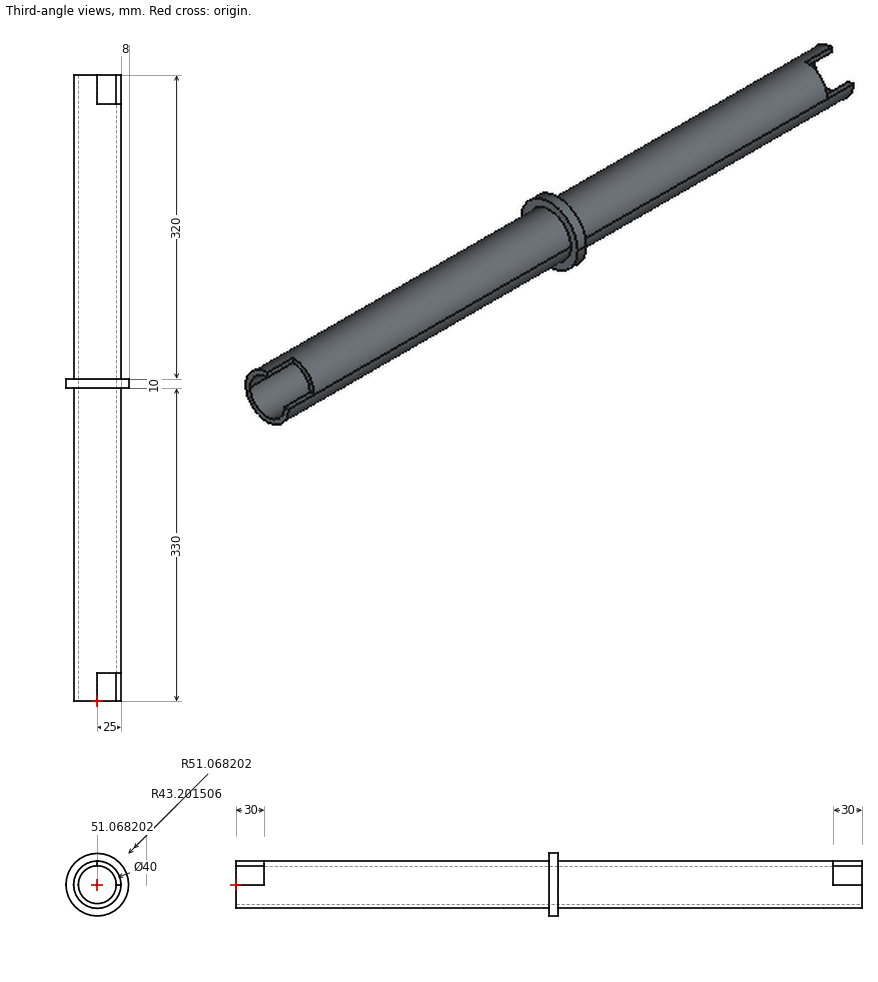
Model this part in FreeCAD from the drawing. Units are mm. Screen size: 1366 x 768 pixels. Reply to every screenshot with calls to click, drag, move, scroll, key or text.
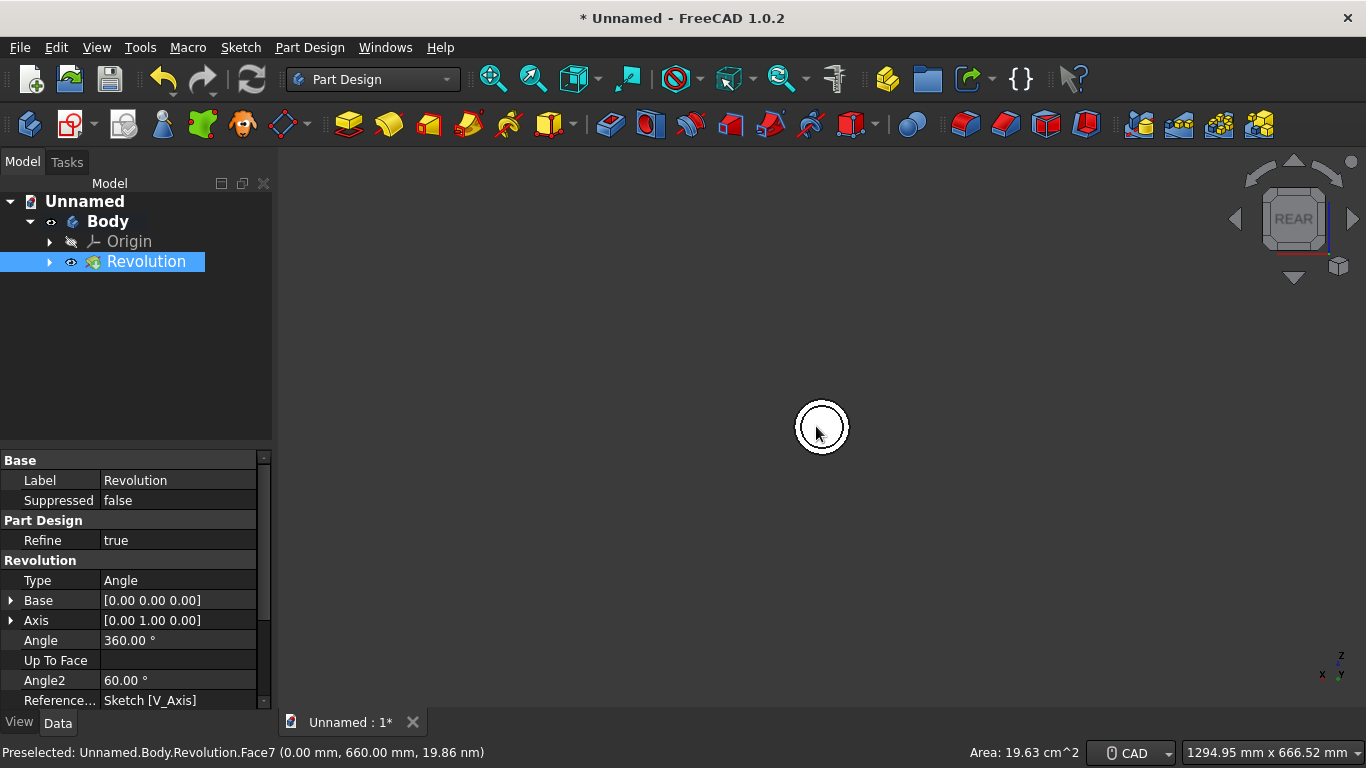
click(70, 124)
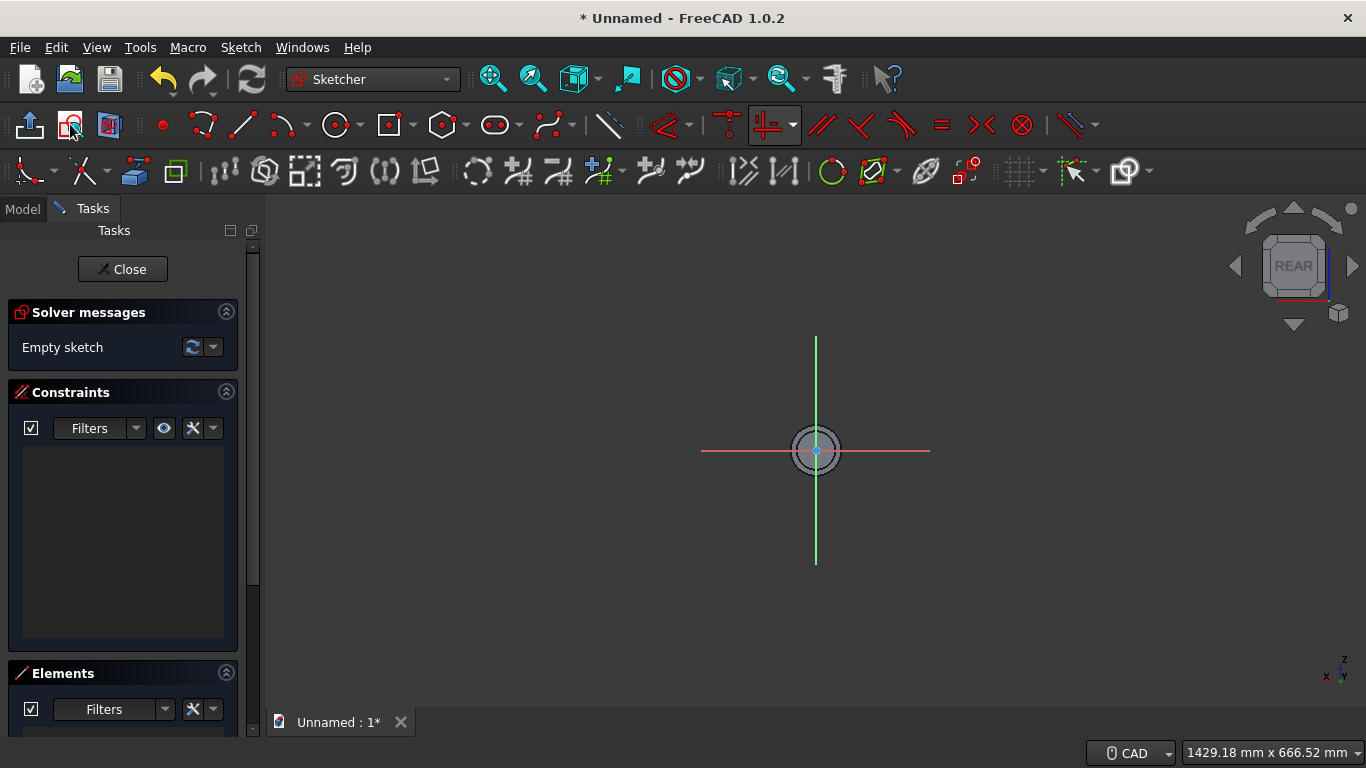
scroll(823, 450, up, 12)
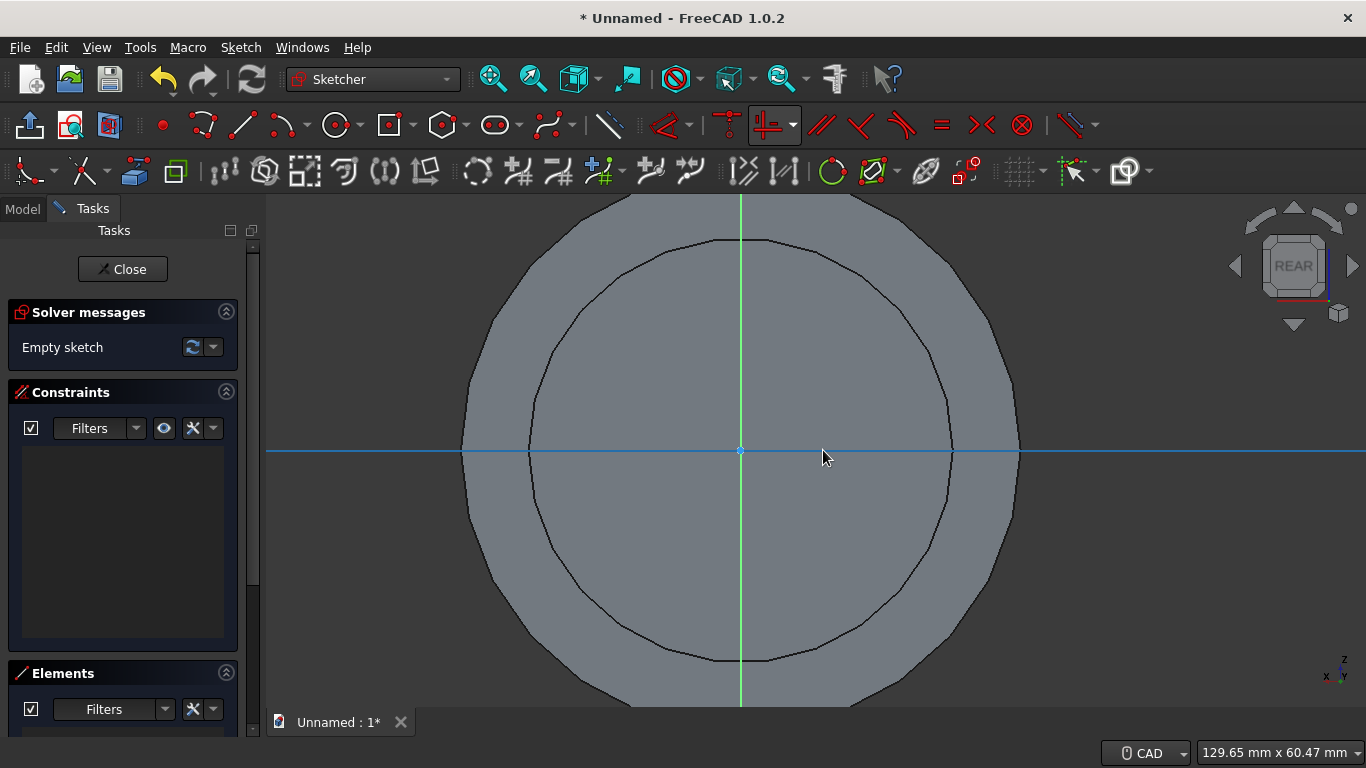
click(336, 126)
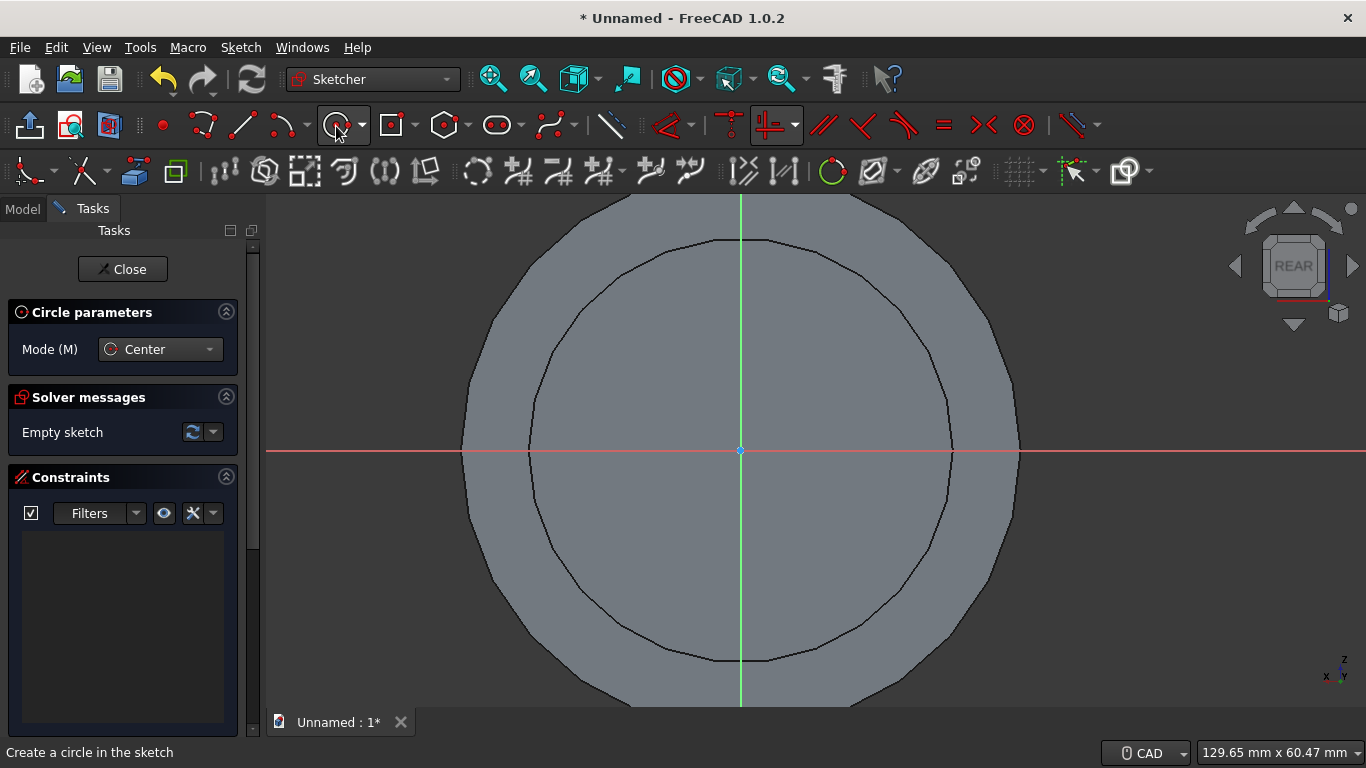
click(741, 450)
move(861, 331)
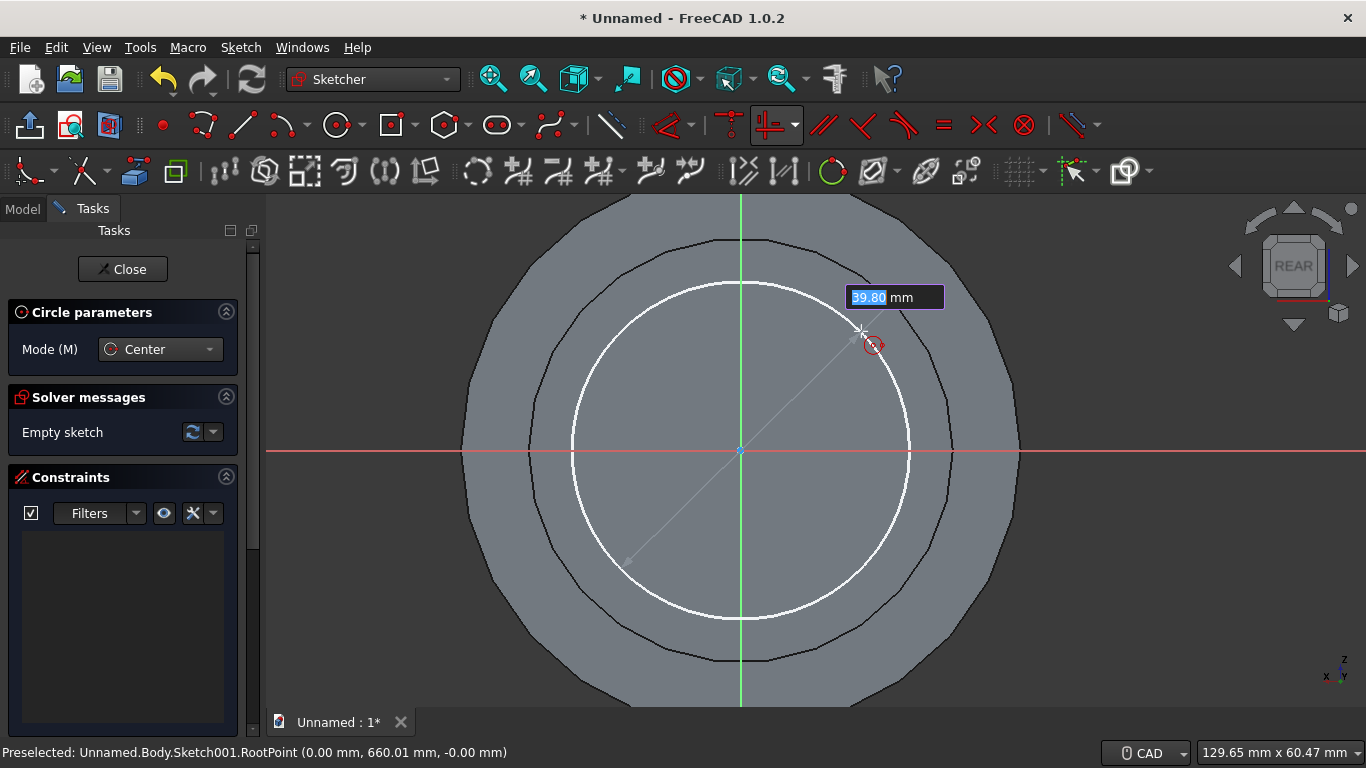
text(40)
key(Return)
key(Escape)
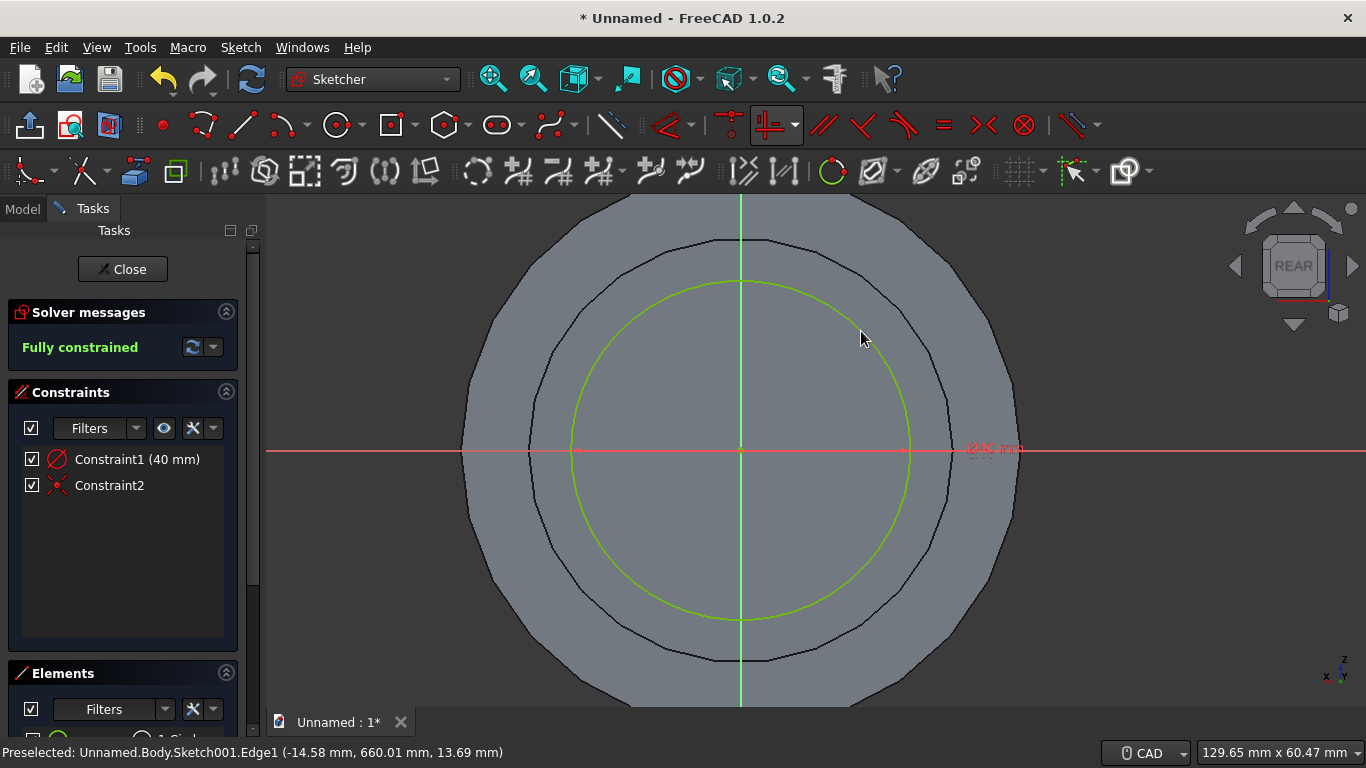
click(123, 269)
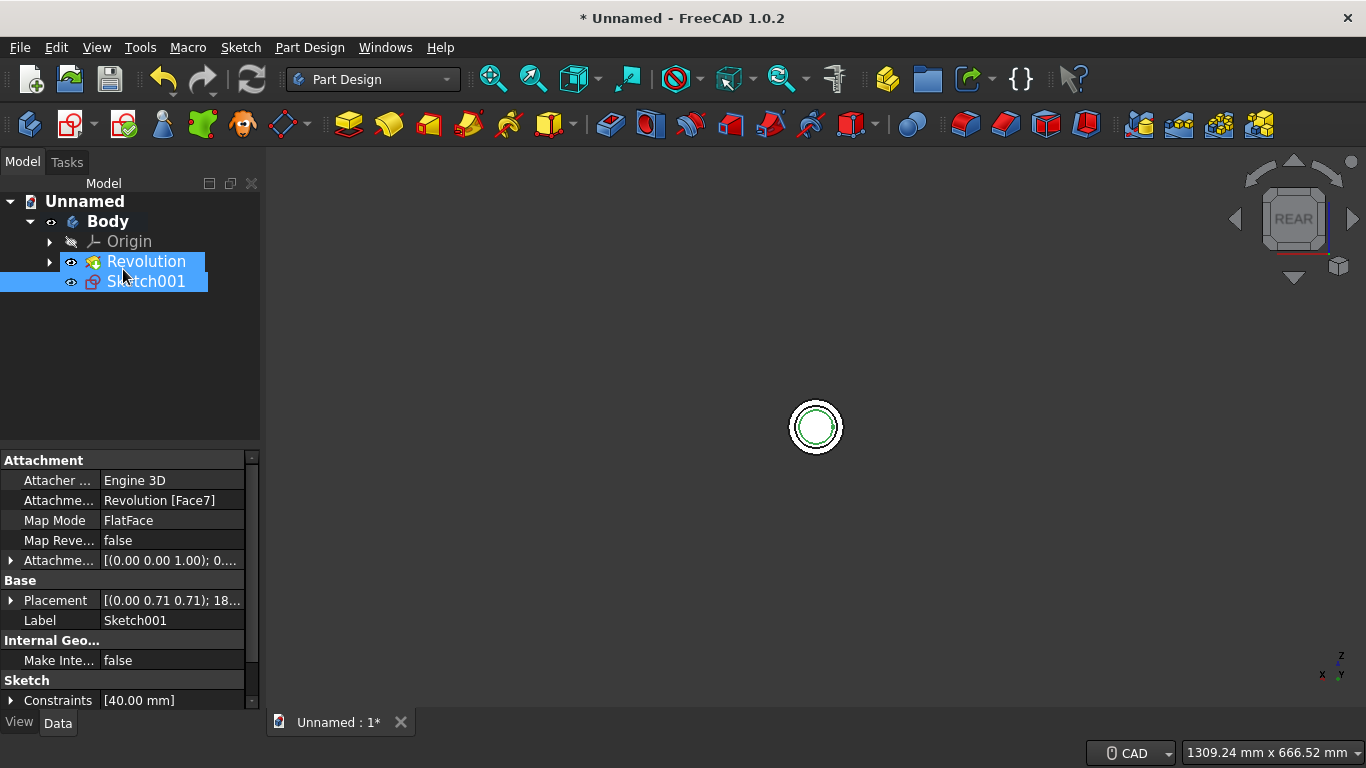
click(612, 124)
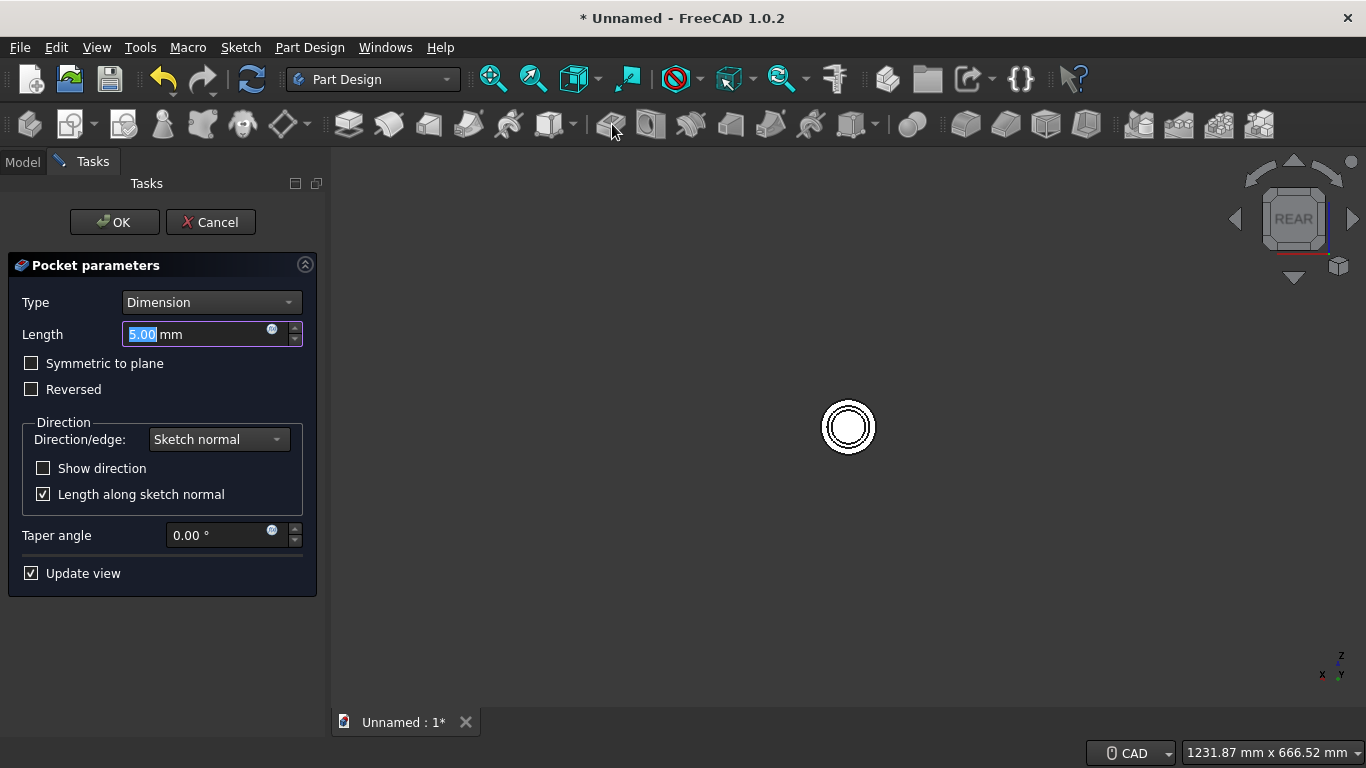
click(212, 302)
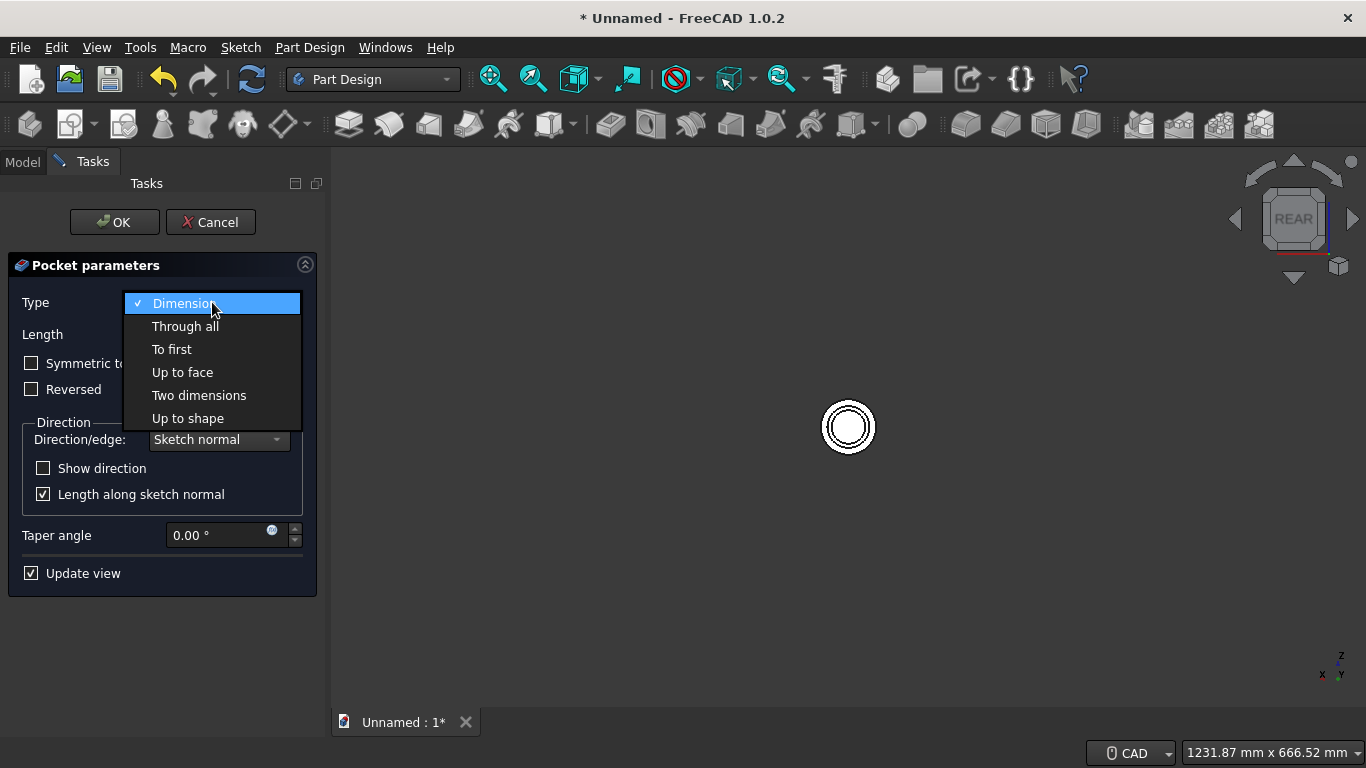
click(212, 350)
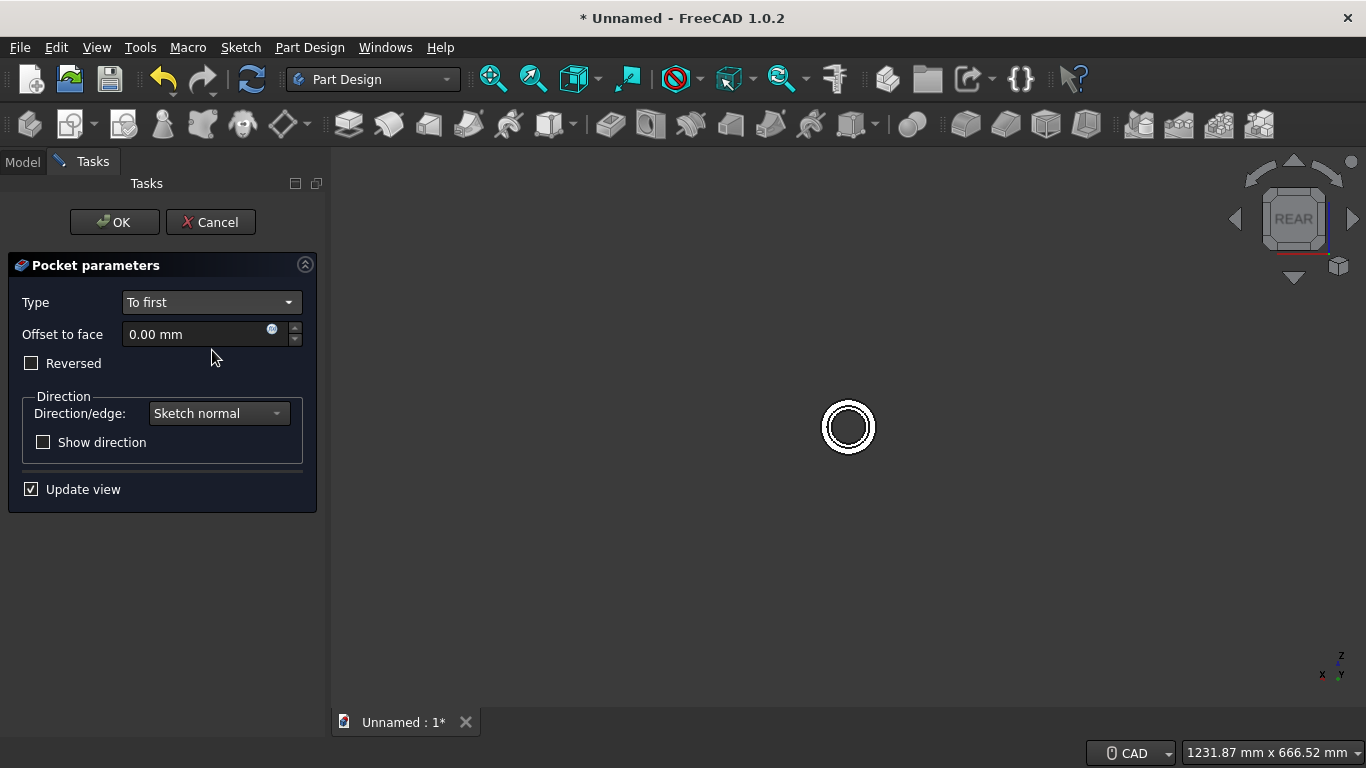
click(115, 222)